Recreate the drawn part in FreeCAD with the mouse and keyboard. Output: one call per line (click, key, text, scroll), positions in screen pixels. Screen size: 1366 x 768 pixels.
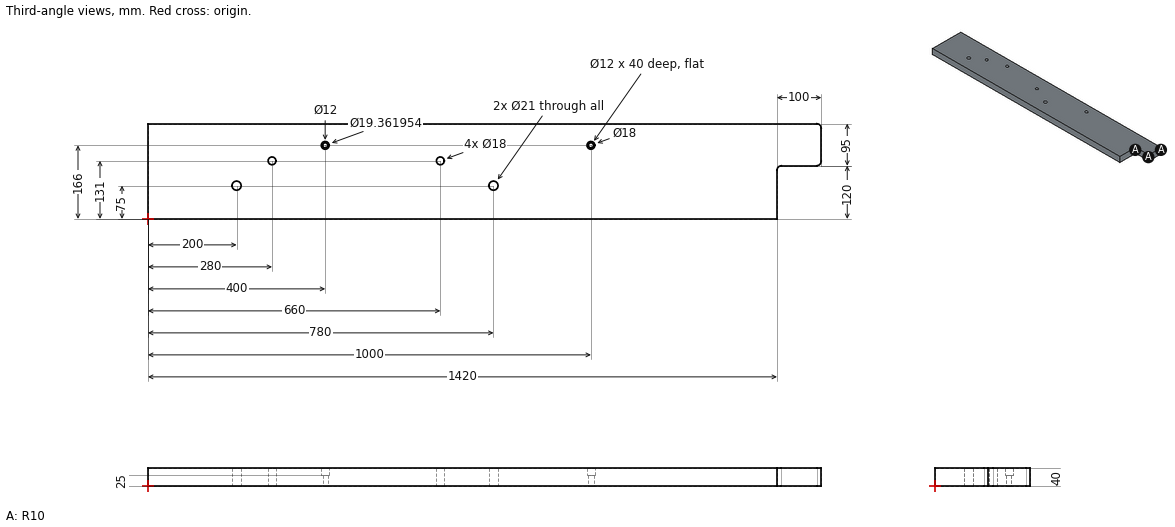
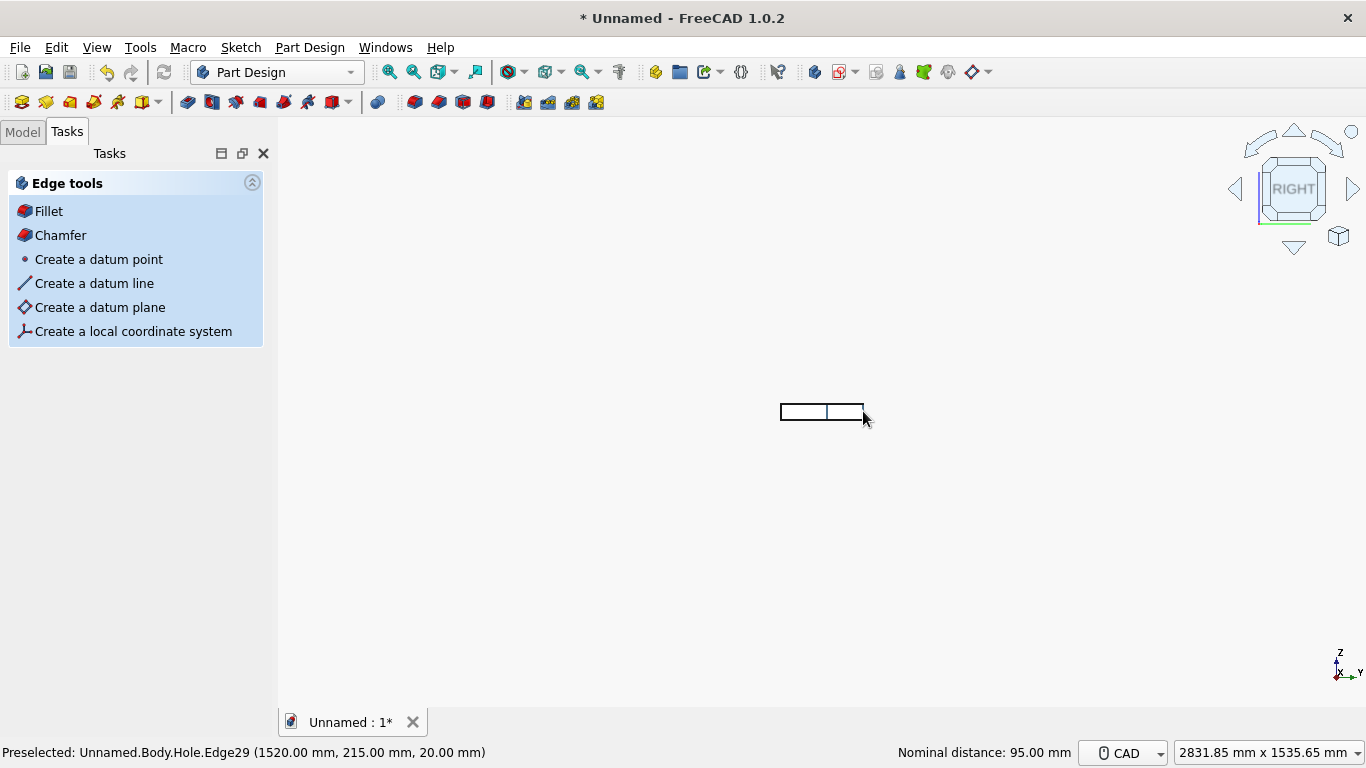
scroll(827, 411, up, 5)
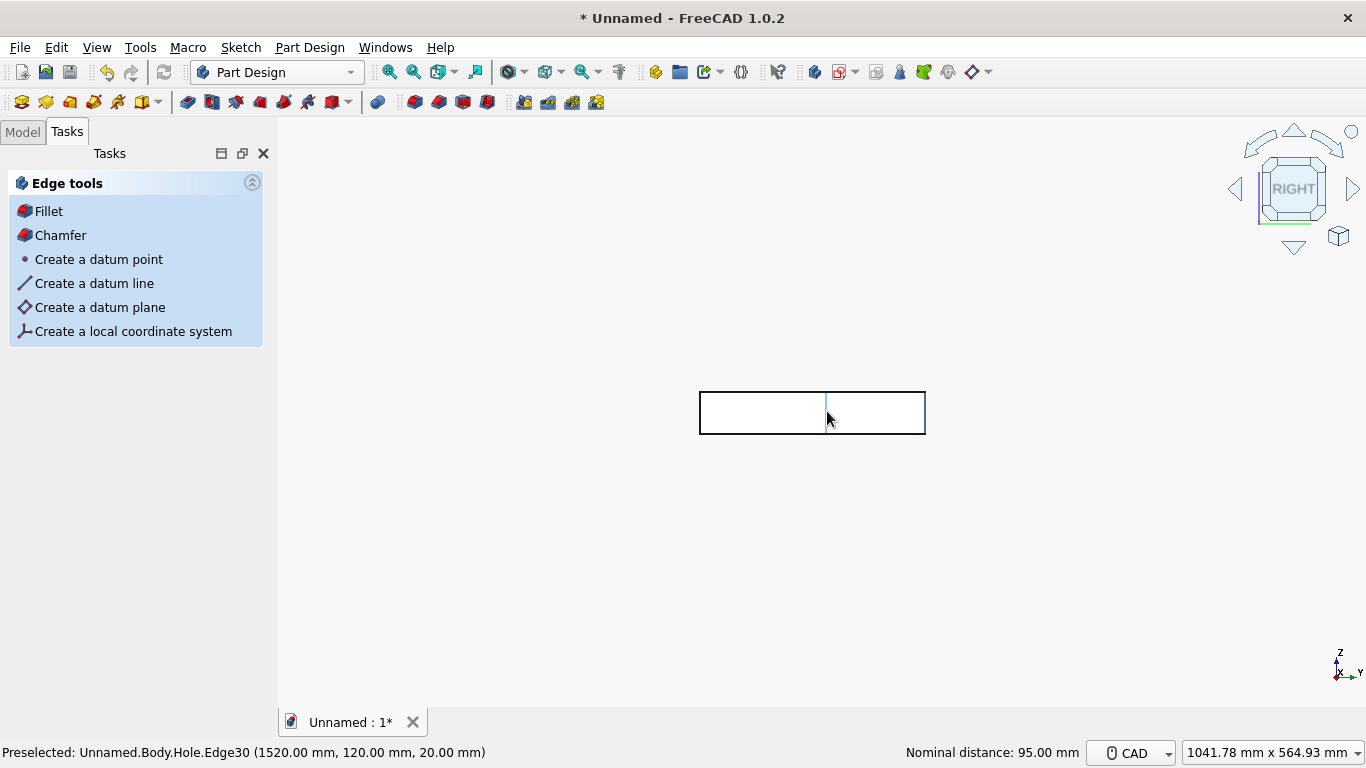
key(v)
key(f)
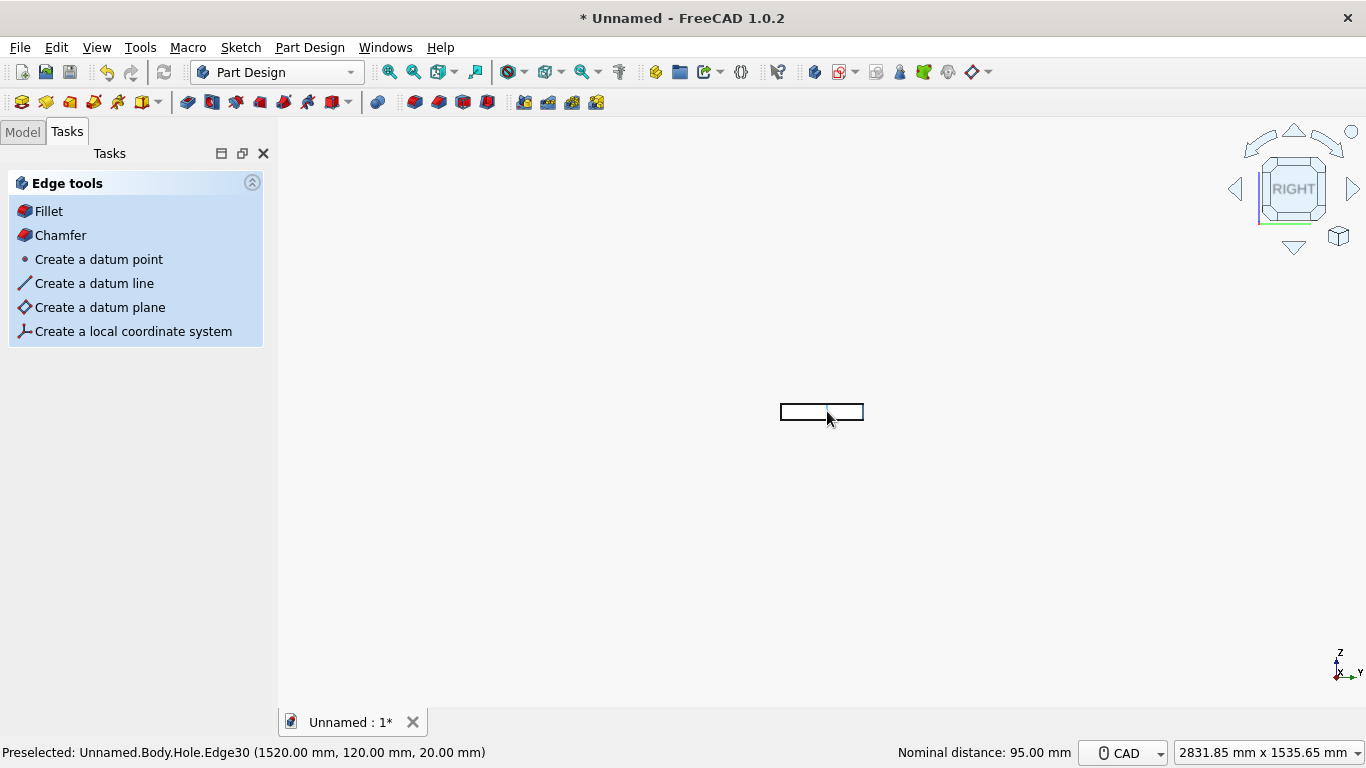
key(5)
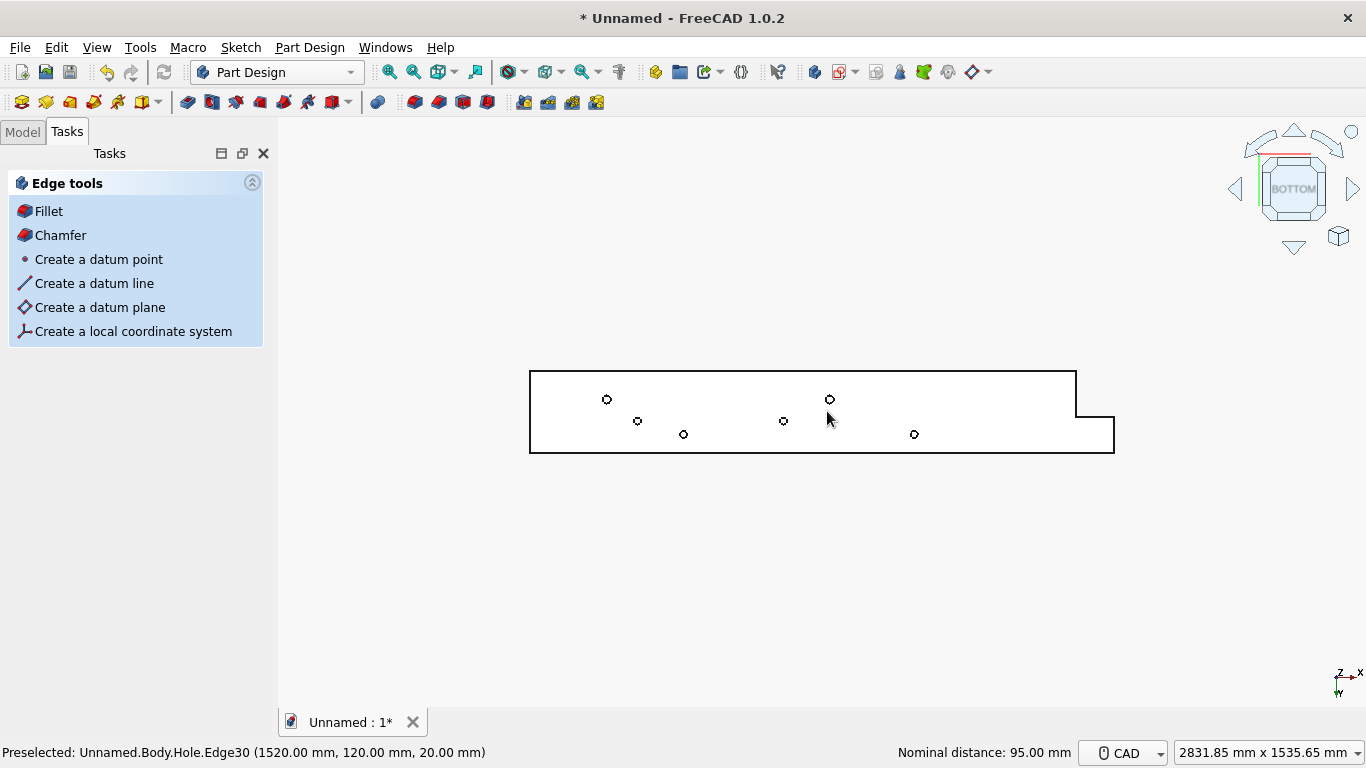
scroll(1076, 416, up, 5)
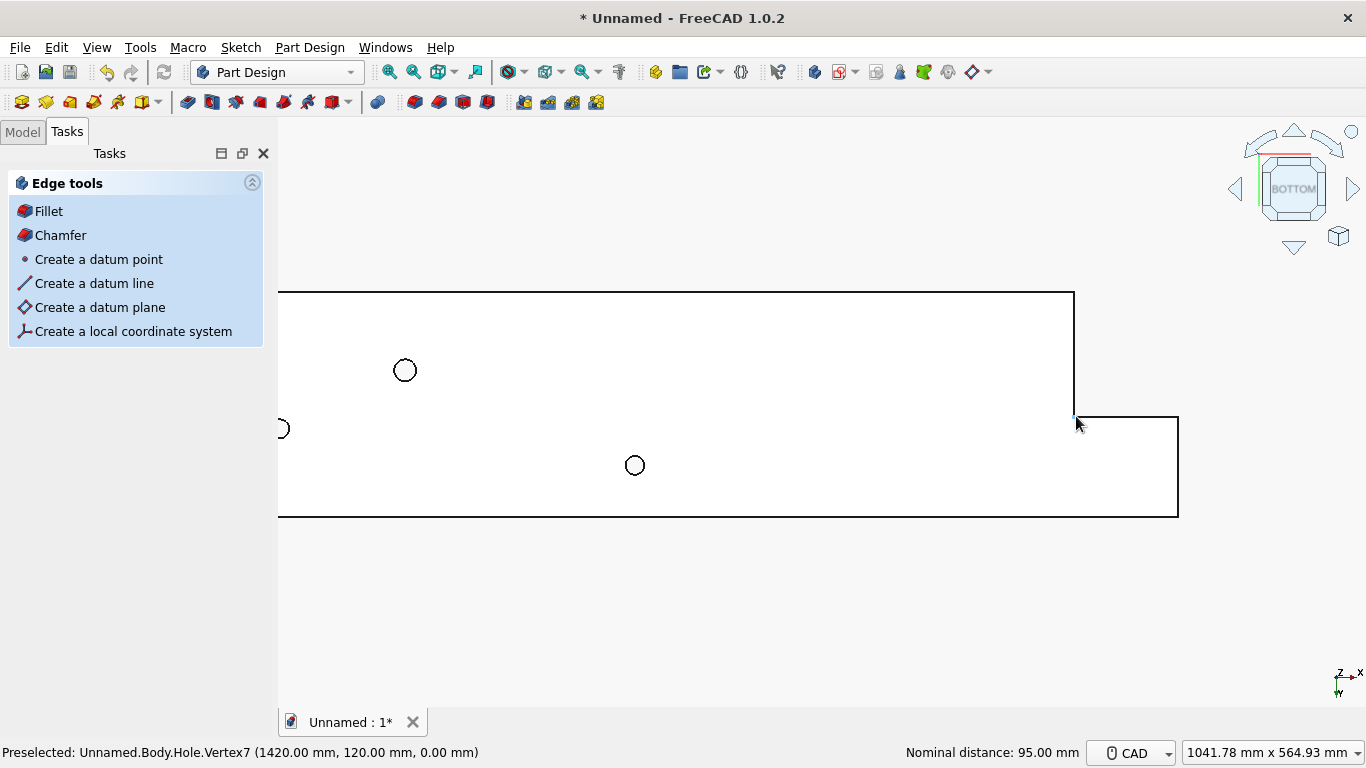
key(v)
key(f)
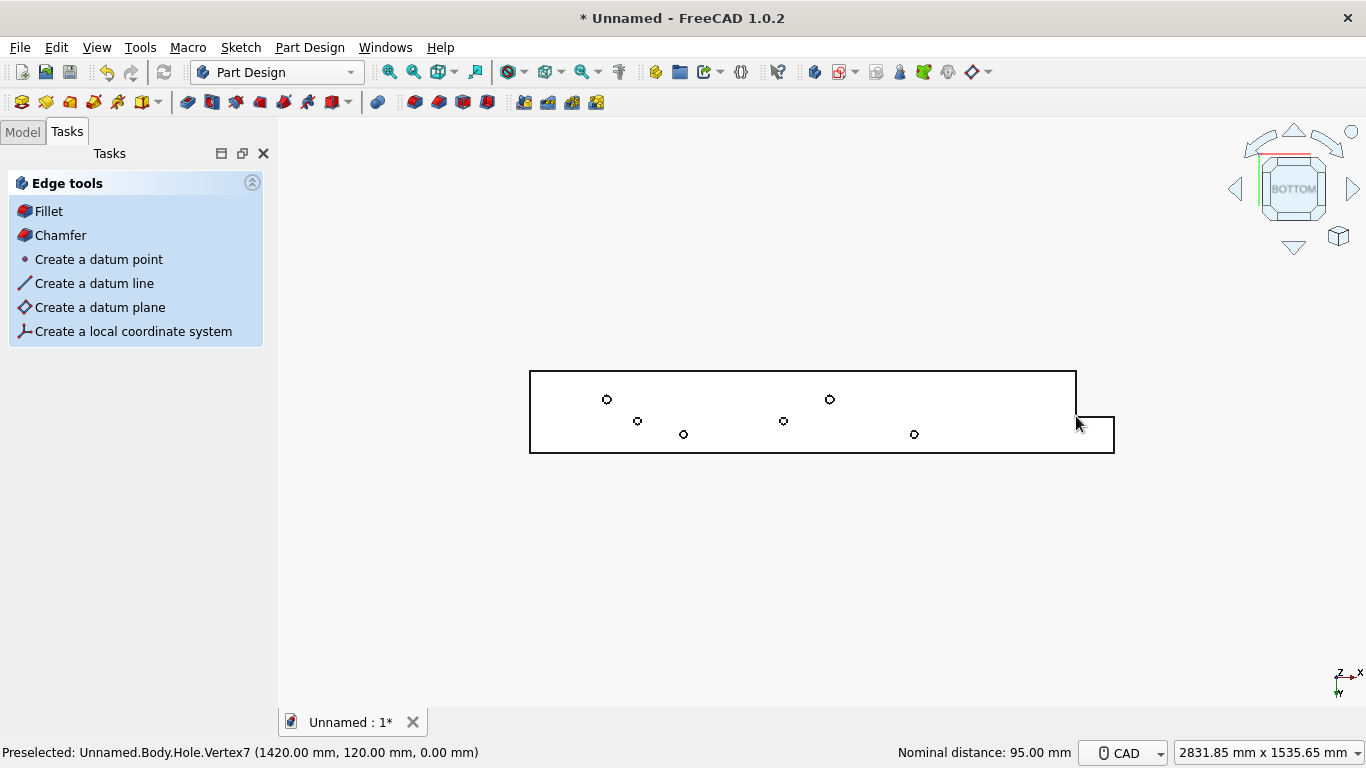
key(4)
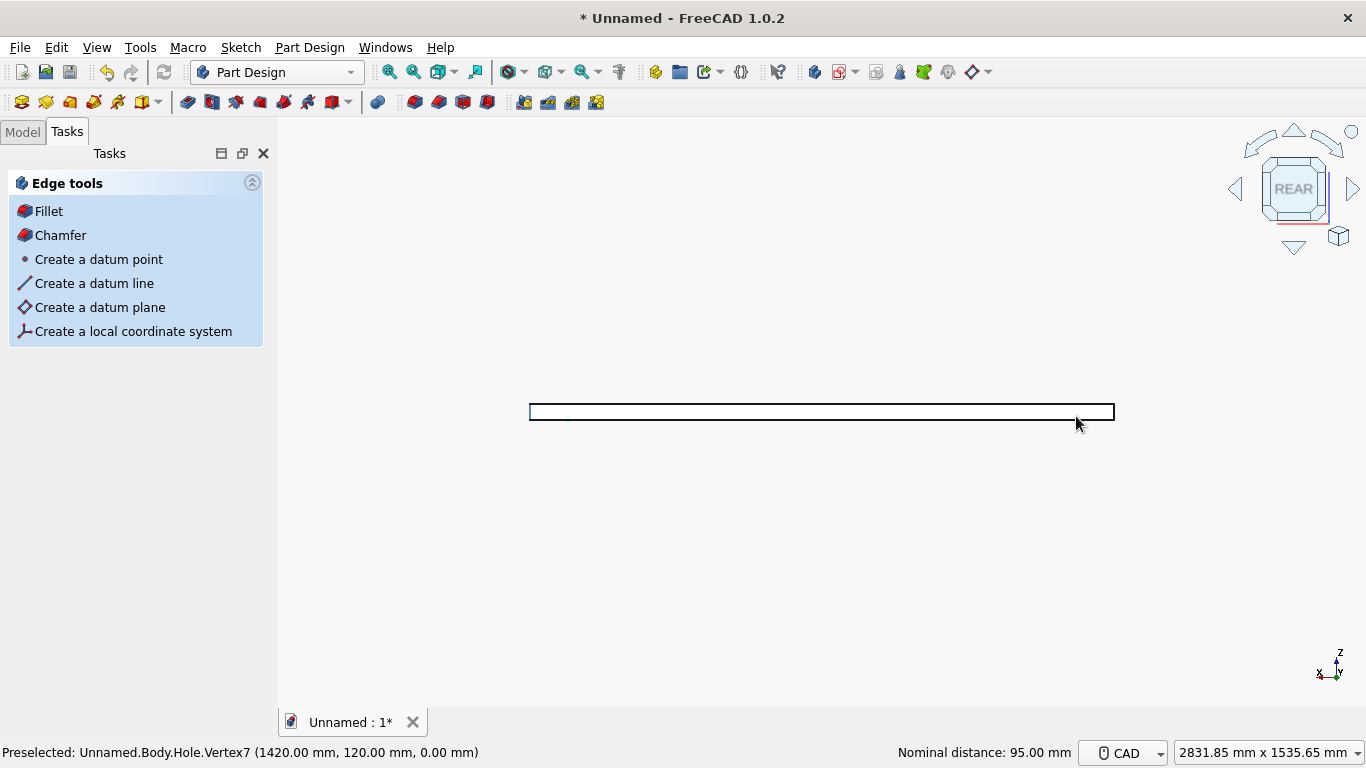
scroll(568, 411, up, 5)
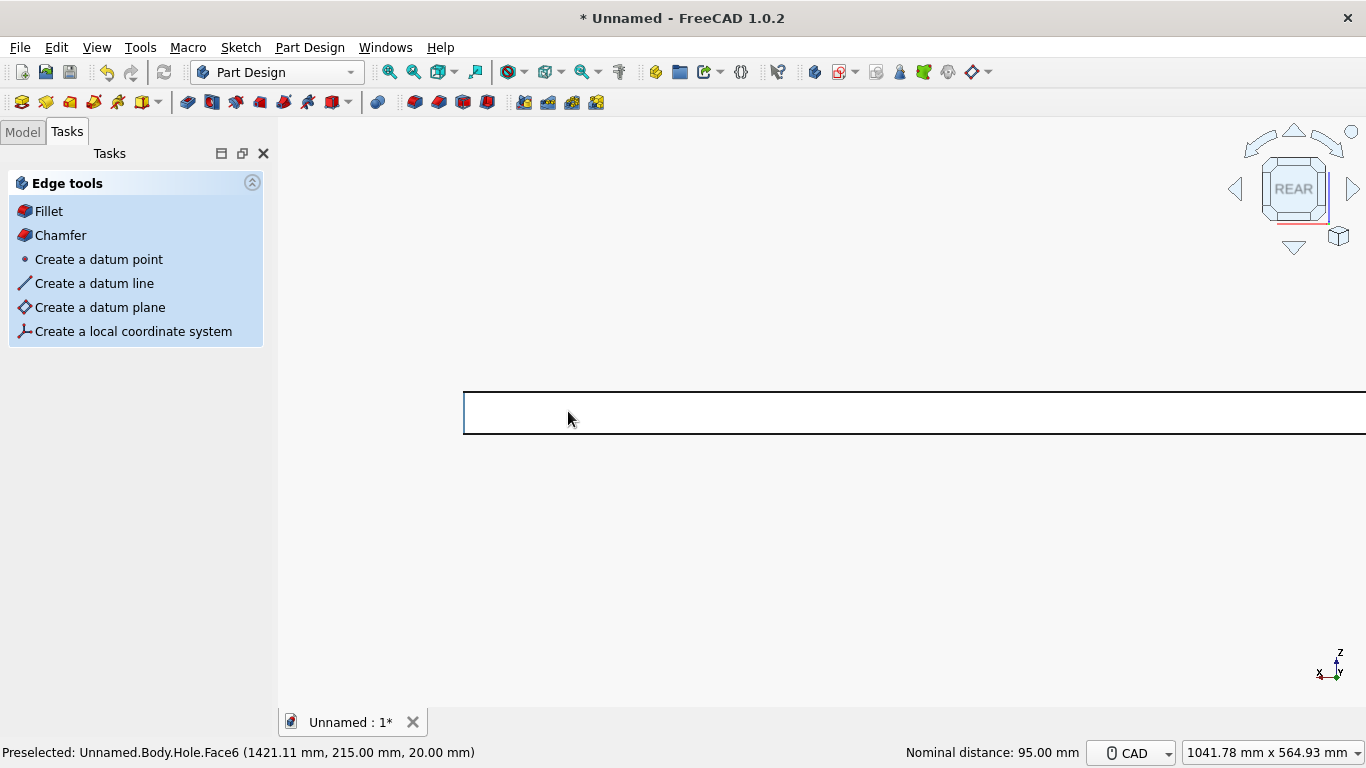
click(390, 72)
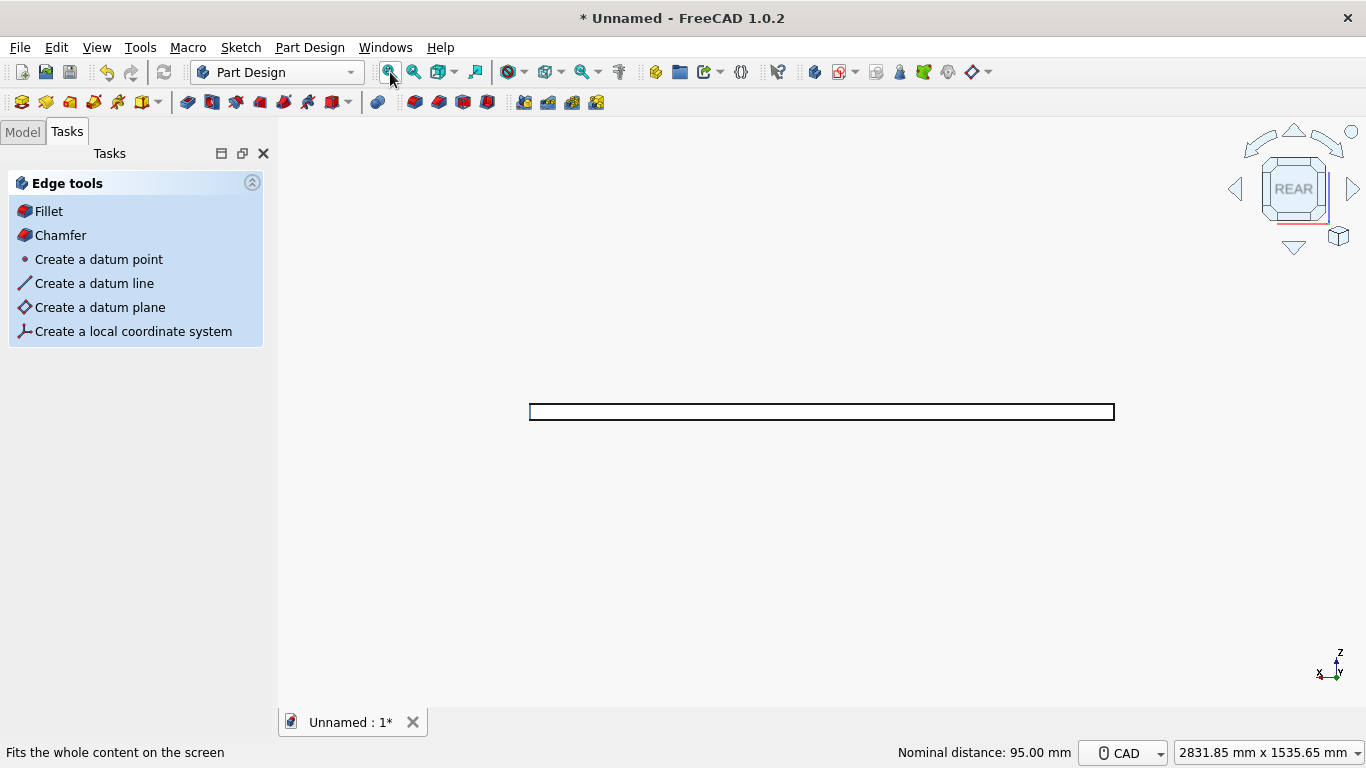
key(6)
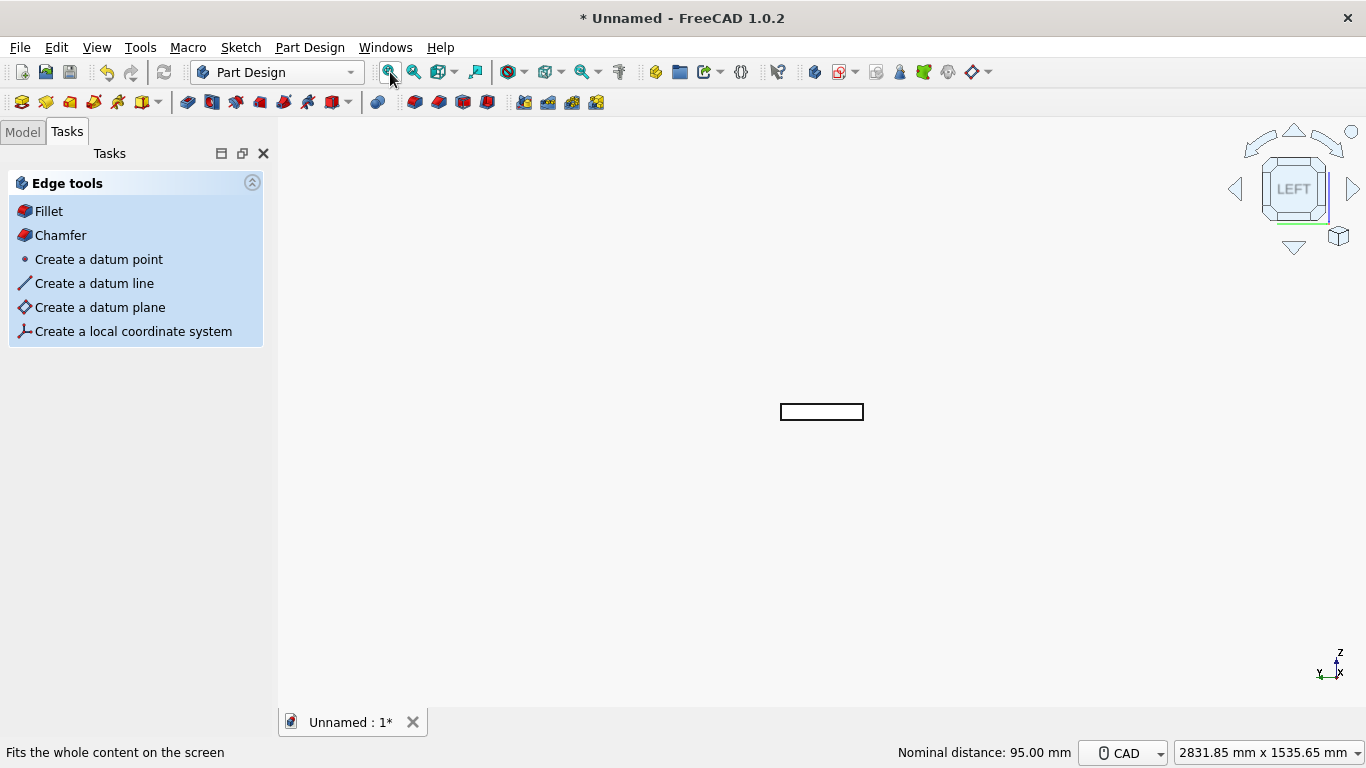
key(v)
key(f)